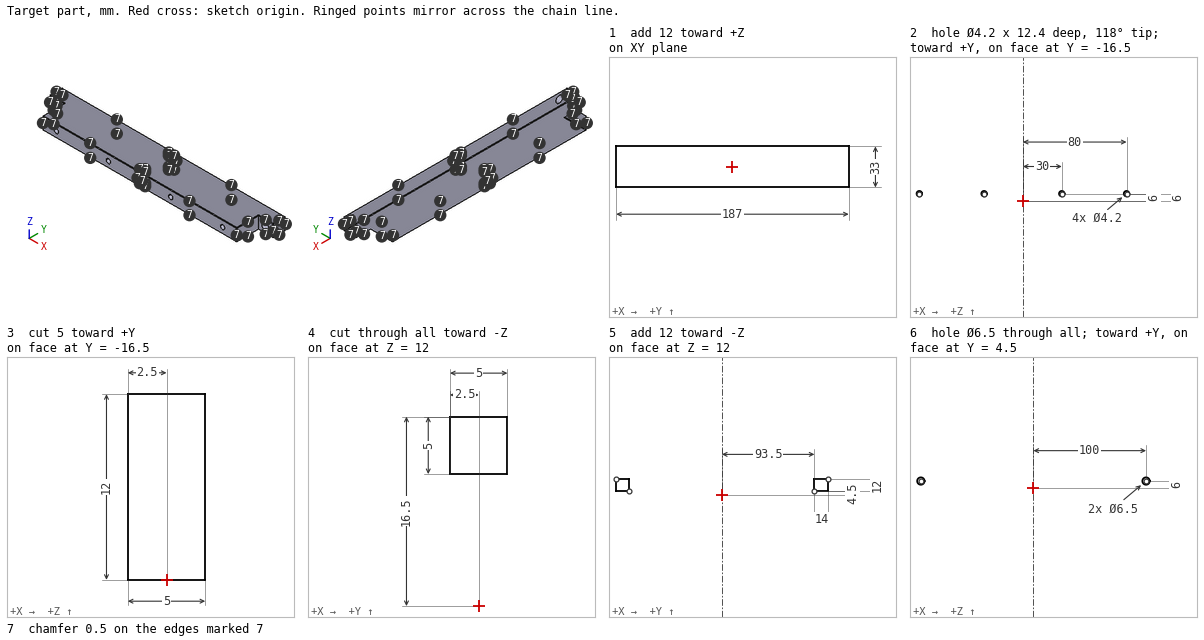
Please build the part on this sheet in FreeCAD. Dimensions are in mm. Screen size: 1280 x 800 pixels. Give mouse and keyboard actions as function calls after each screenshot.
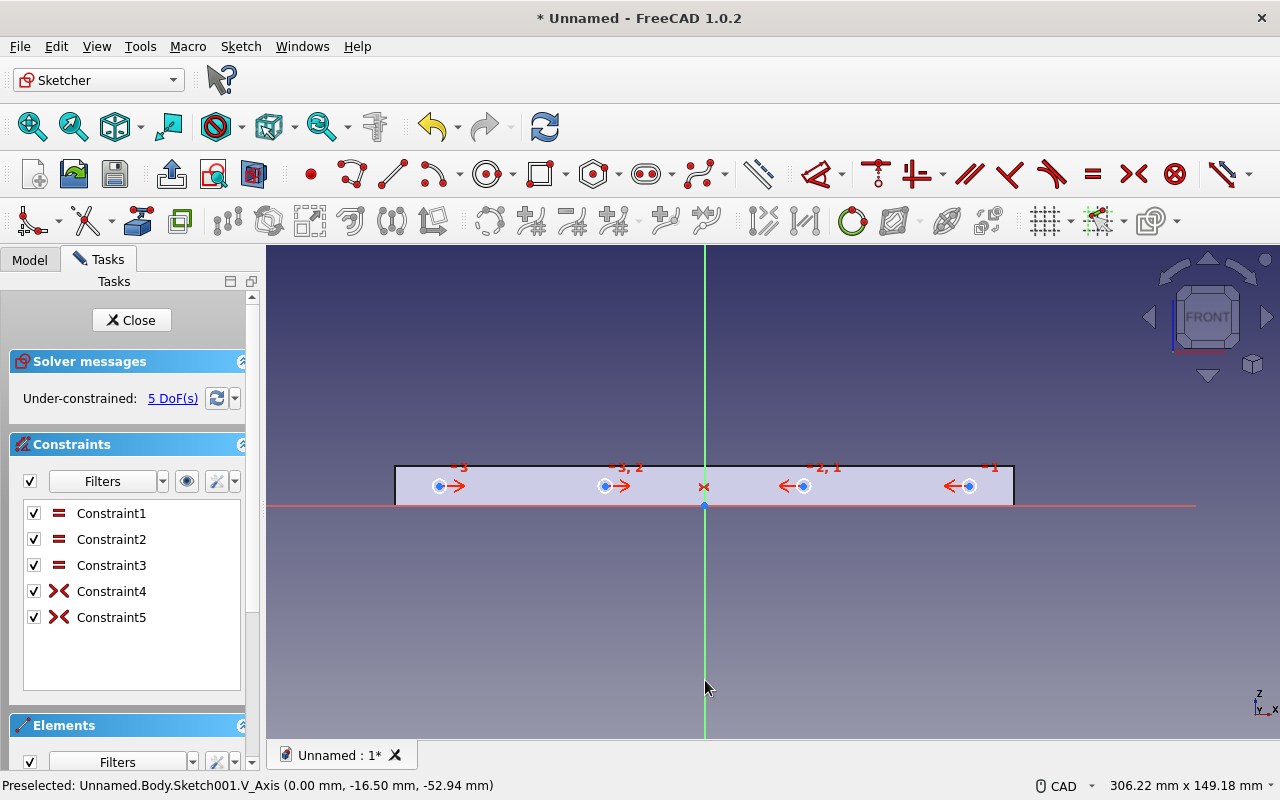
scroll(970, 479, up, 6)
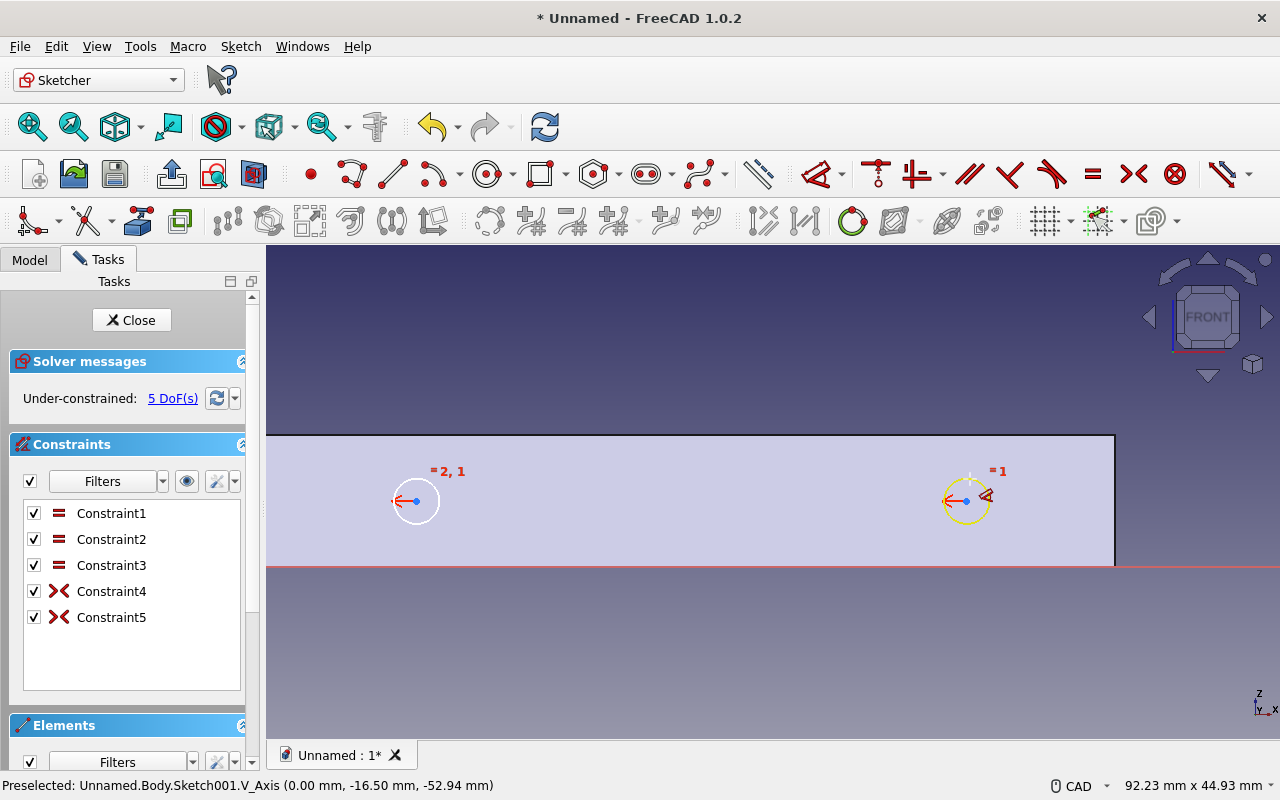
click(967, 479)
click(967, 447)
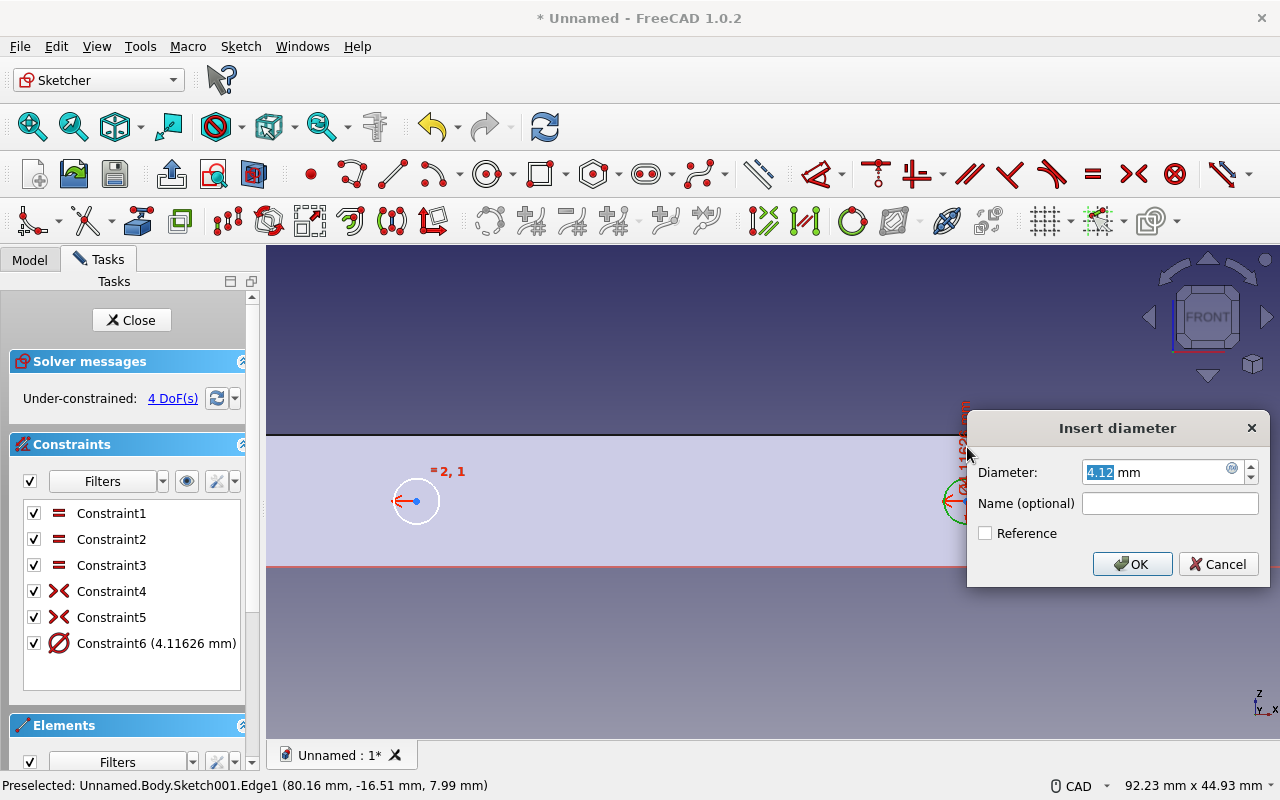
text(4.2)
key(Return)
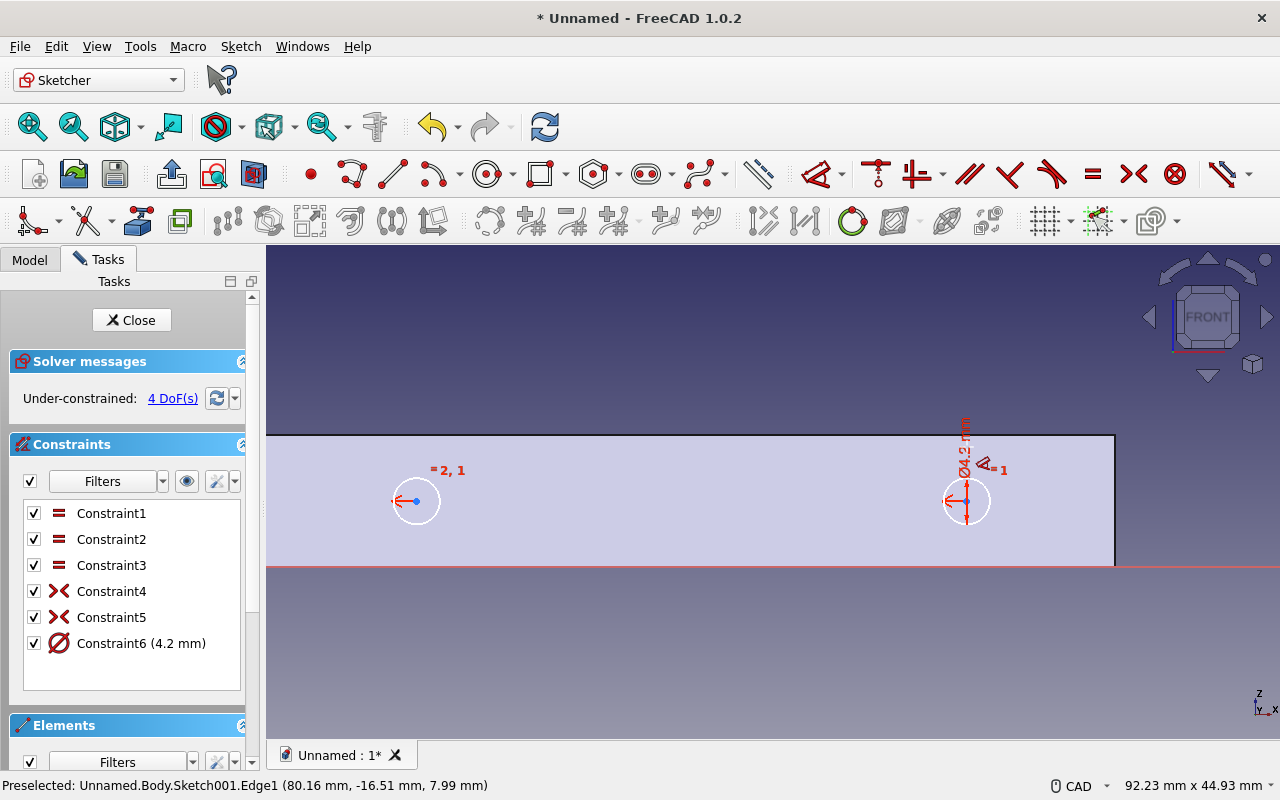
click(967, 501)
click(1001, 534)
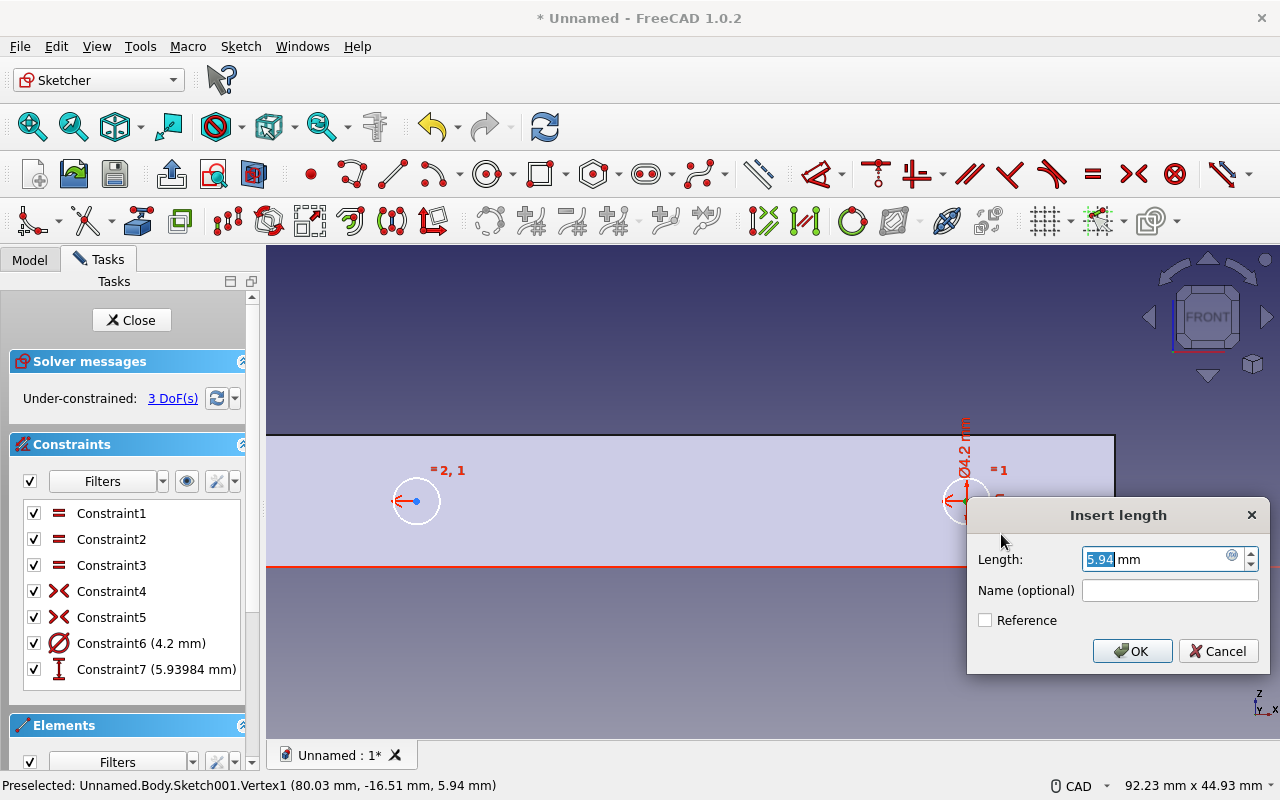
text(6)
key(Return)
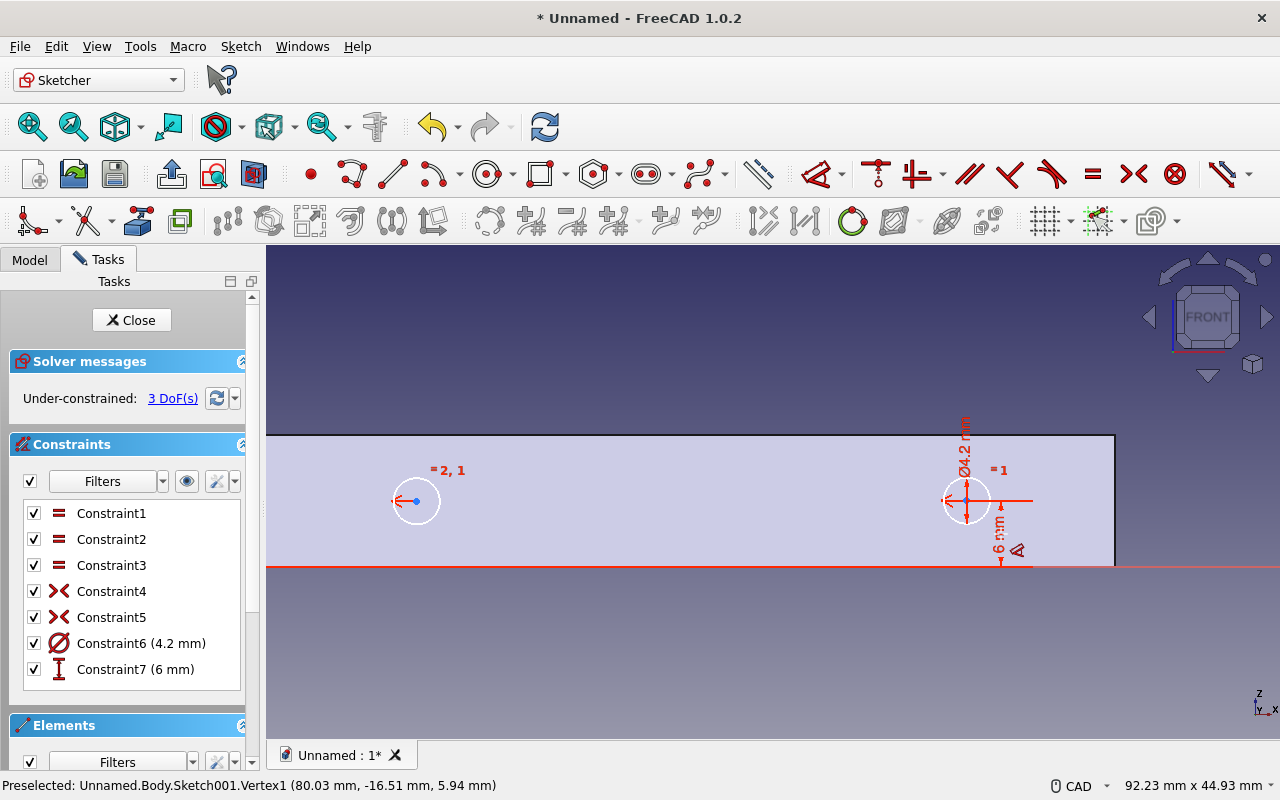
click(417, 501)
click(451, 534)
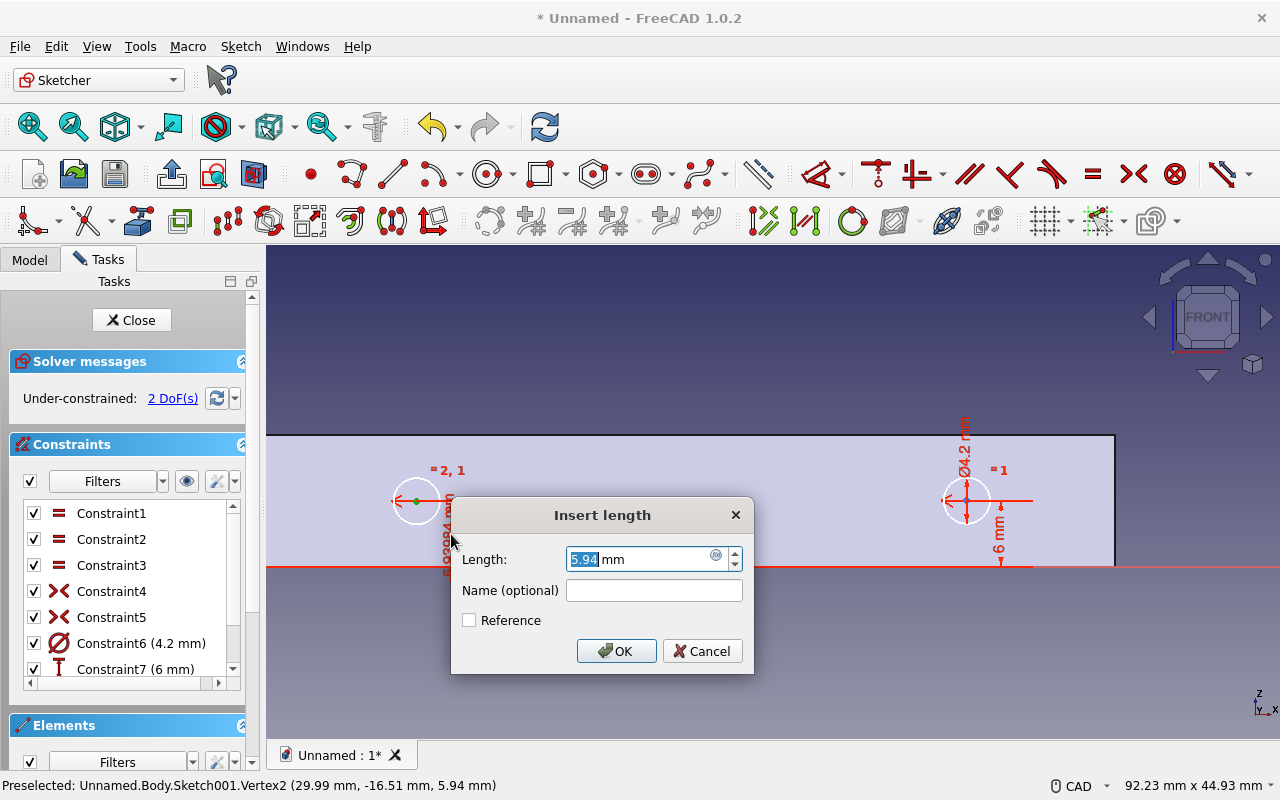
text(6)
key(Return)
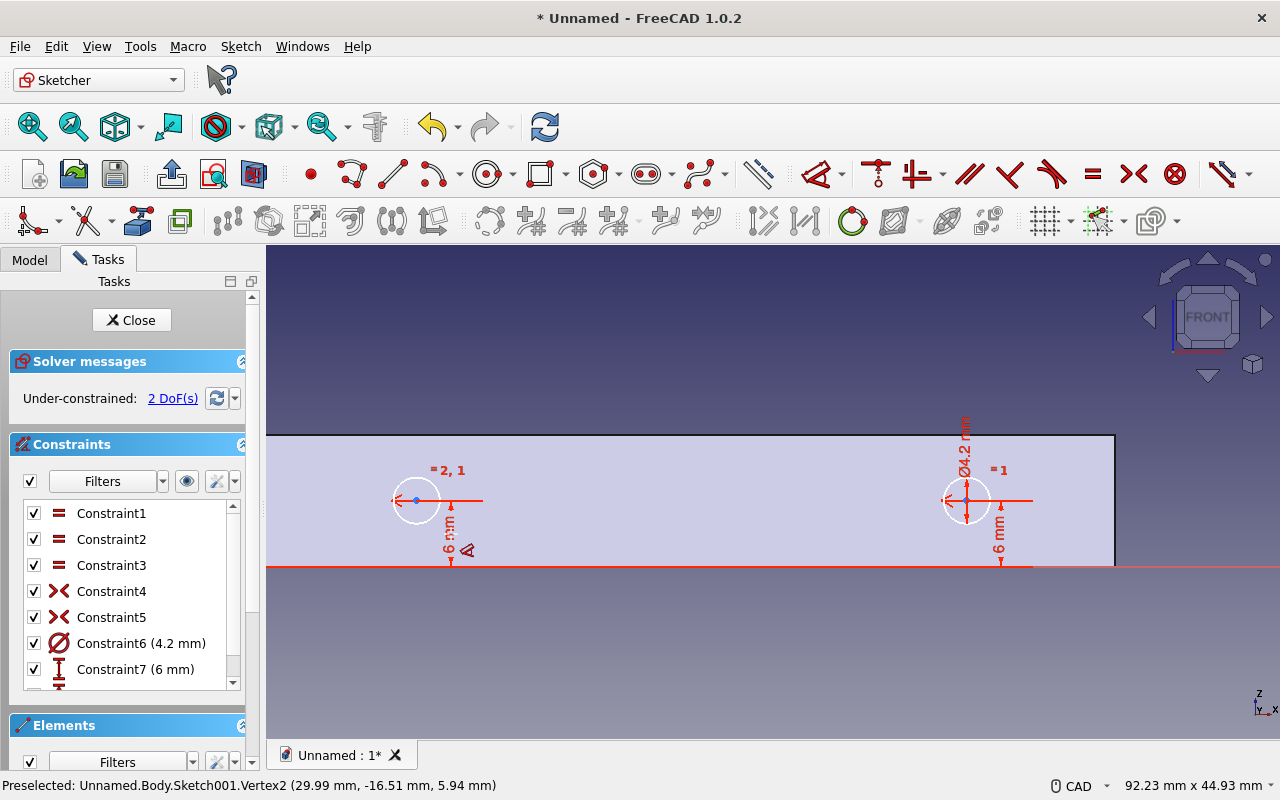
click(967, 501)
click(630, 601)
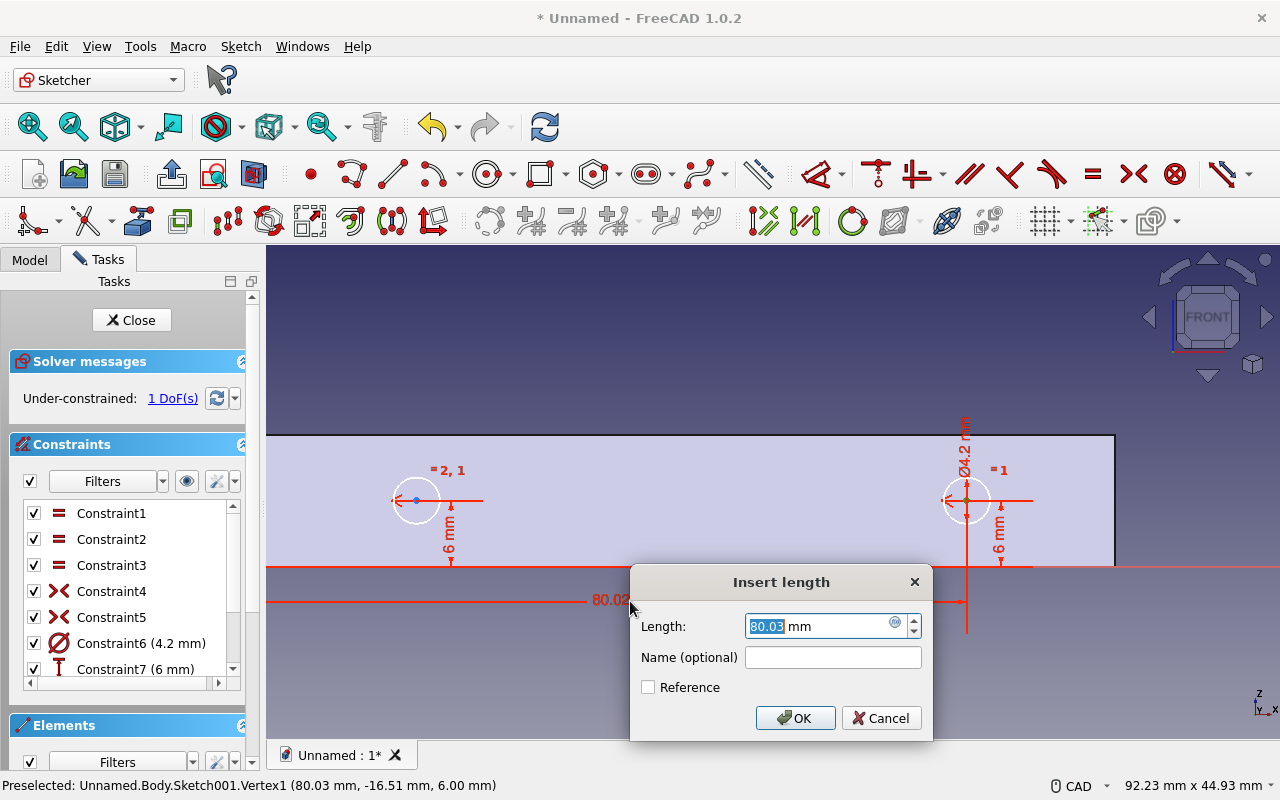
text(80)
key(Return)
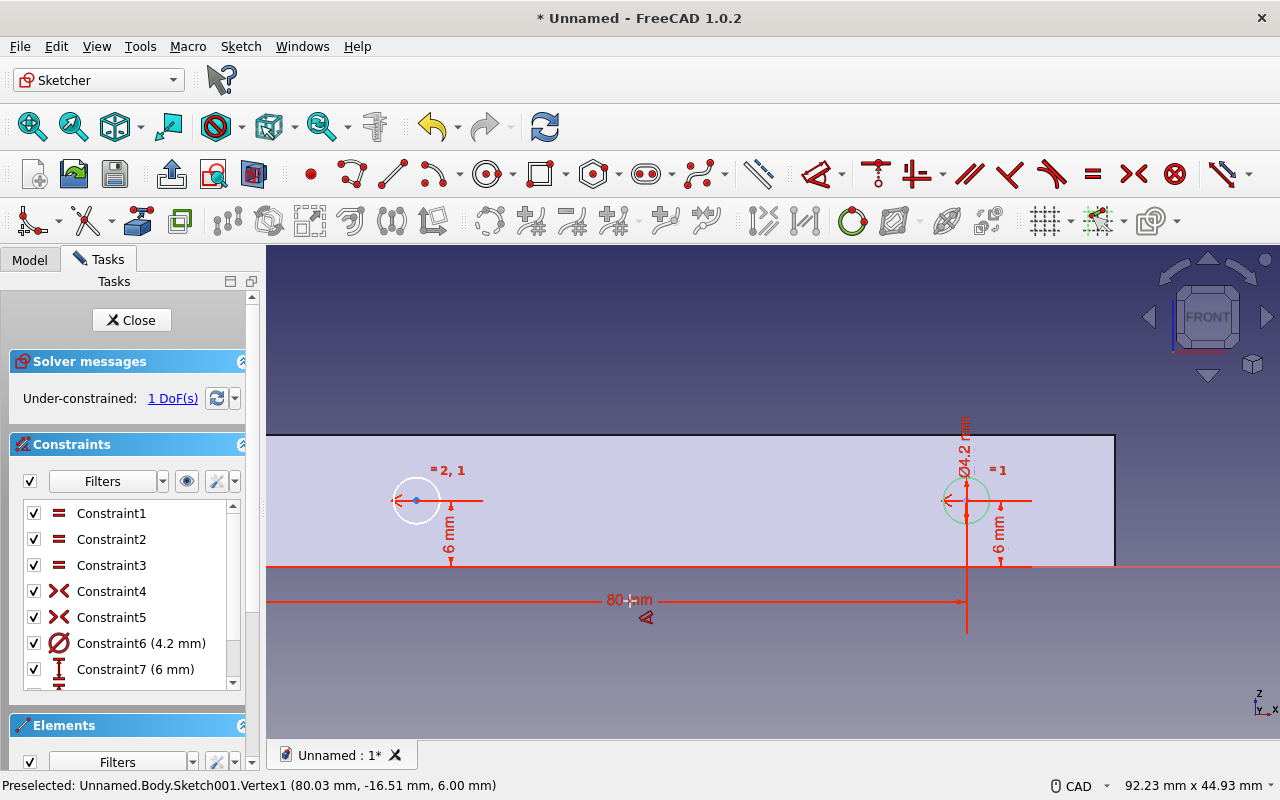
click(417, 501)
click(355, 601)